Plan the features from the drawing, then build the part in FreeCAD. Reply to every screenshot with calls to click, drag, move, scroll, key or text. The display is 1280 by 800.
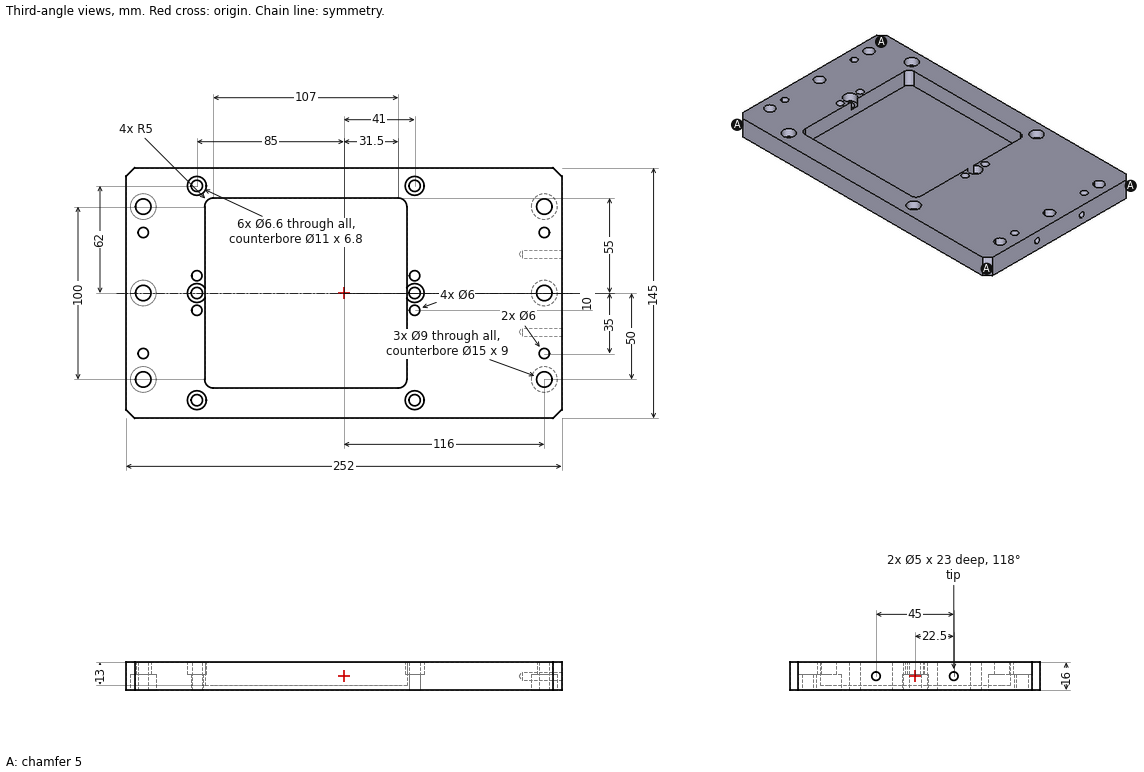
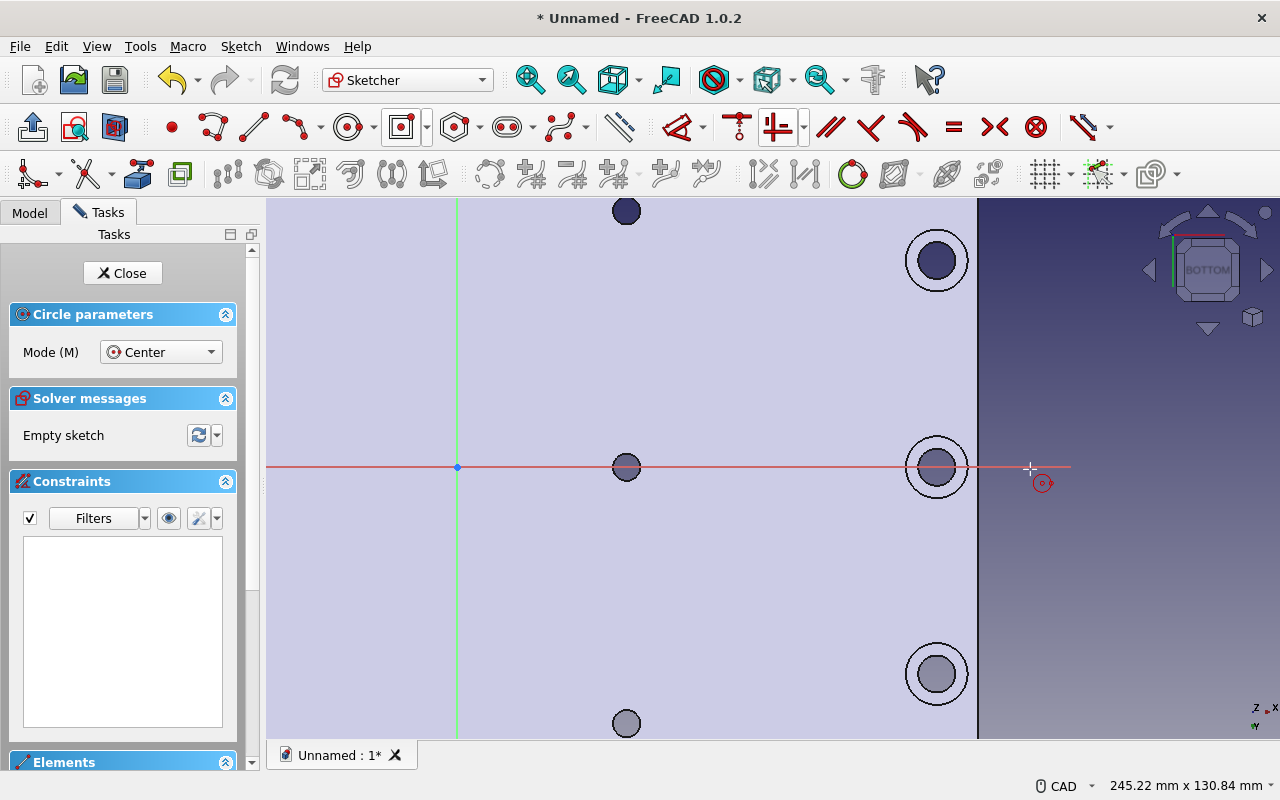
scroll(937, 323, up, 4)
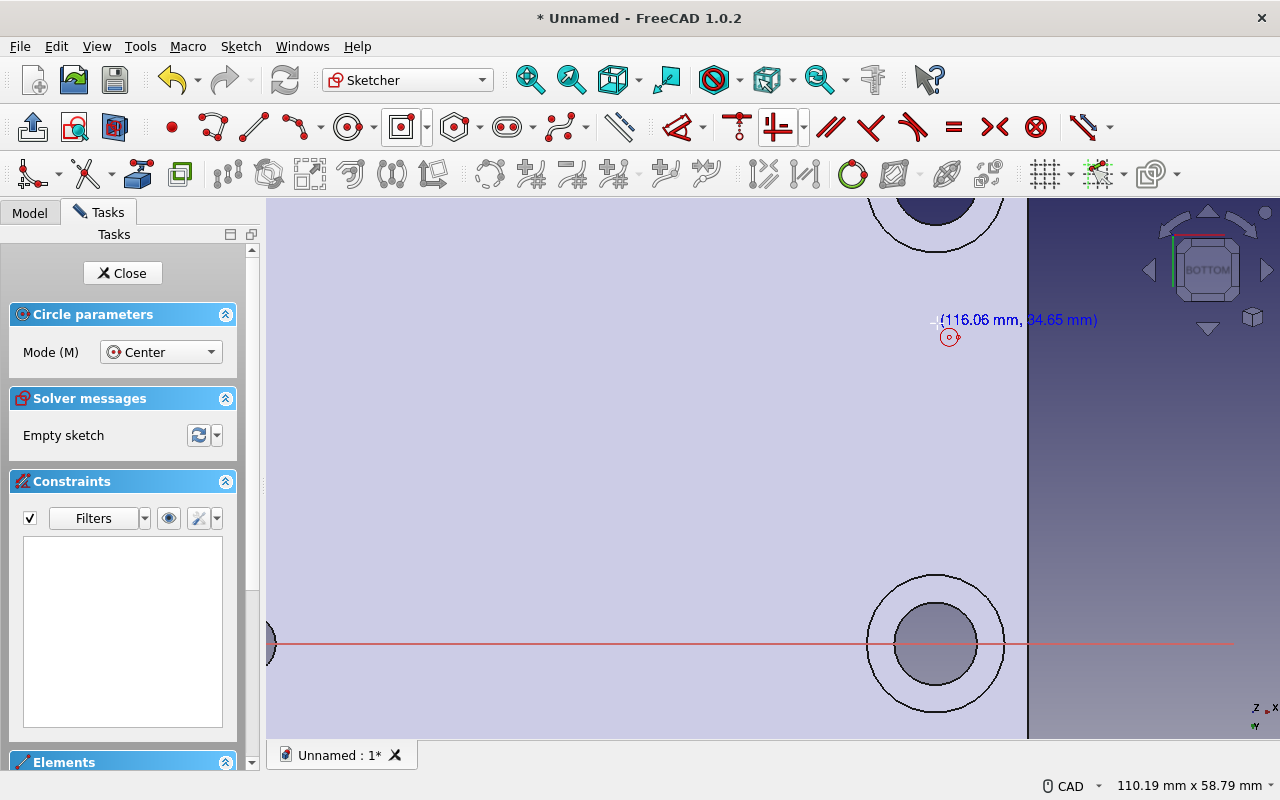
click(936, 322)
move(955, 302)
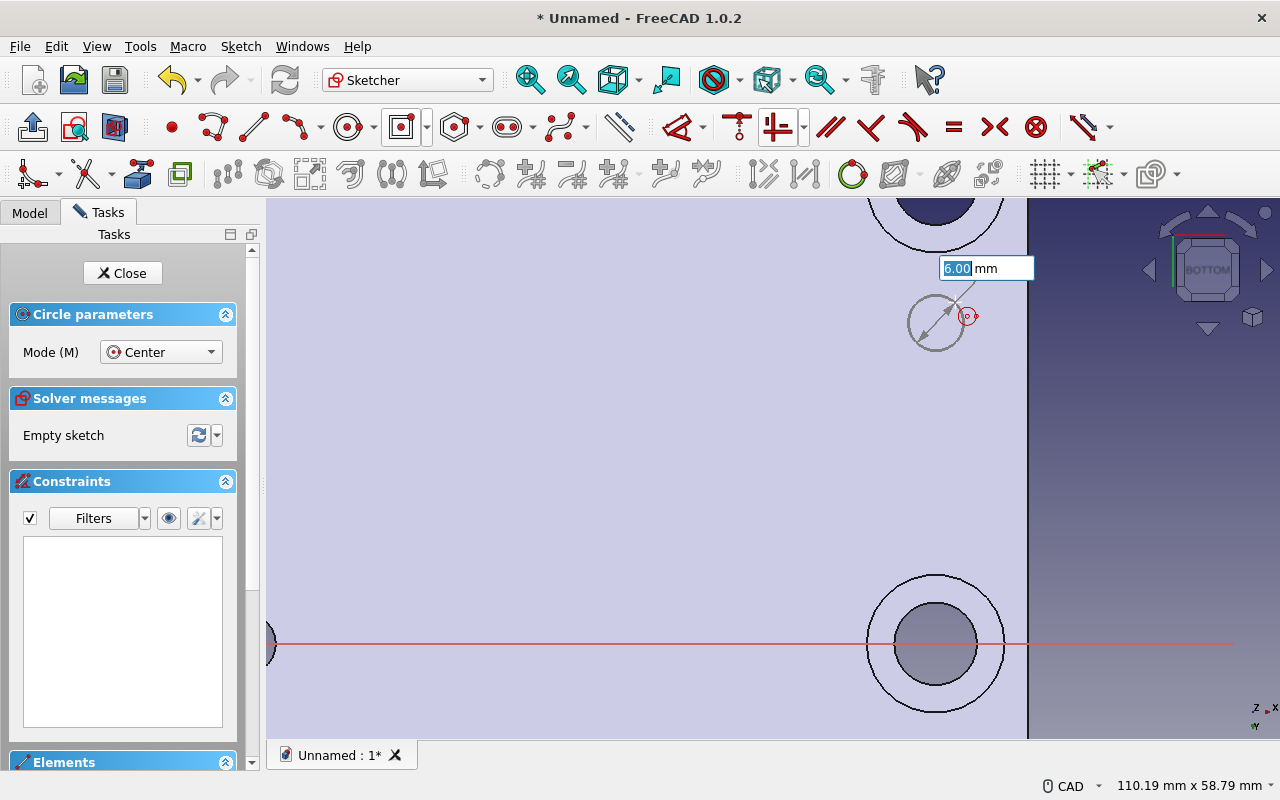
text(6)
key(Return)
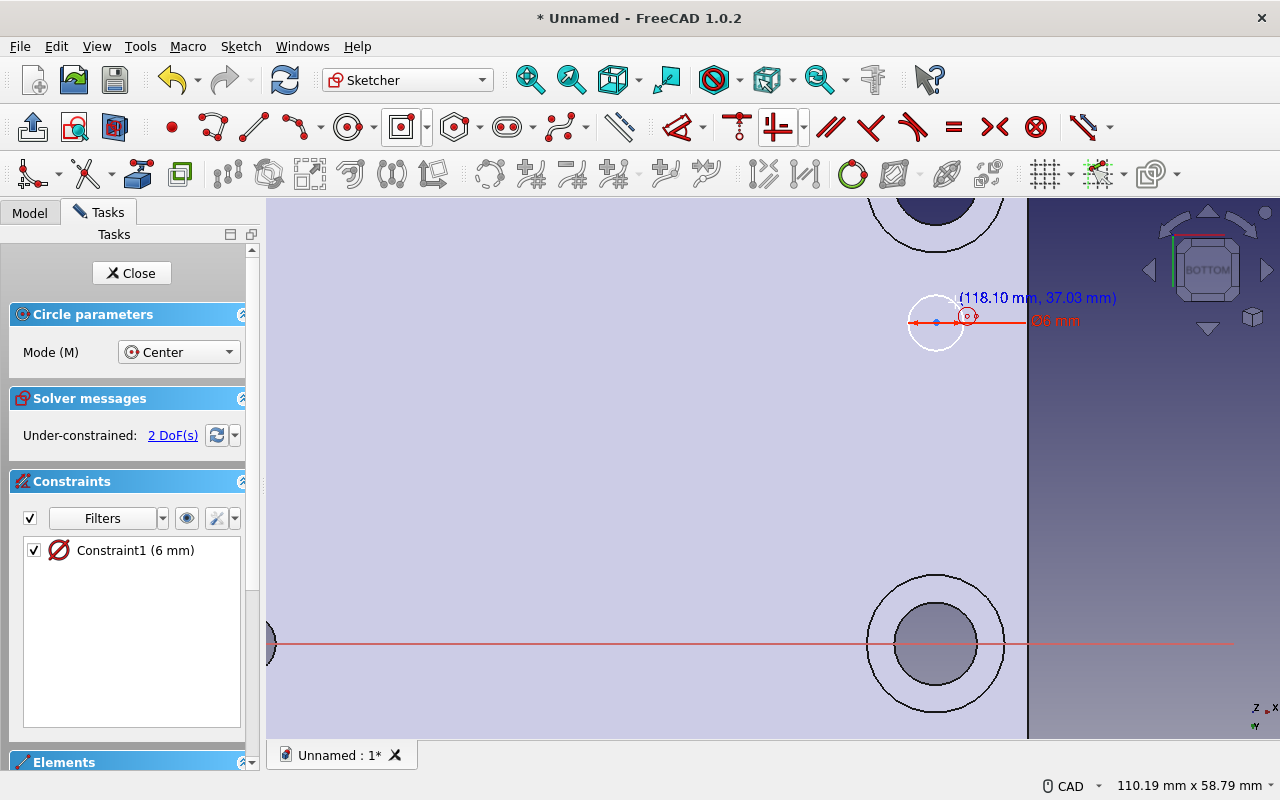
scroll(940, 325, down, 4)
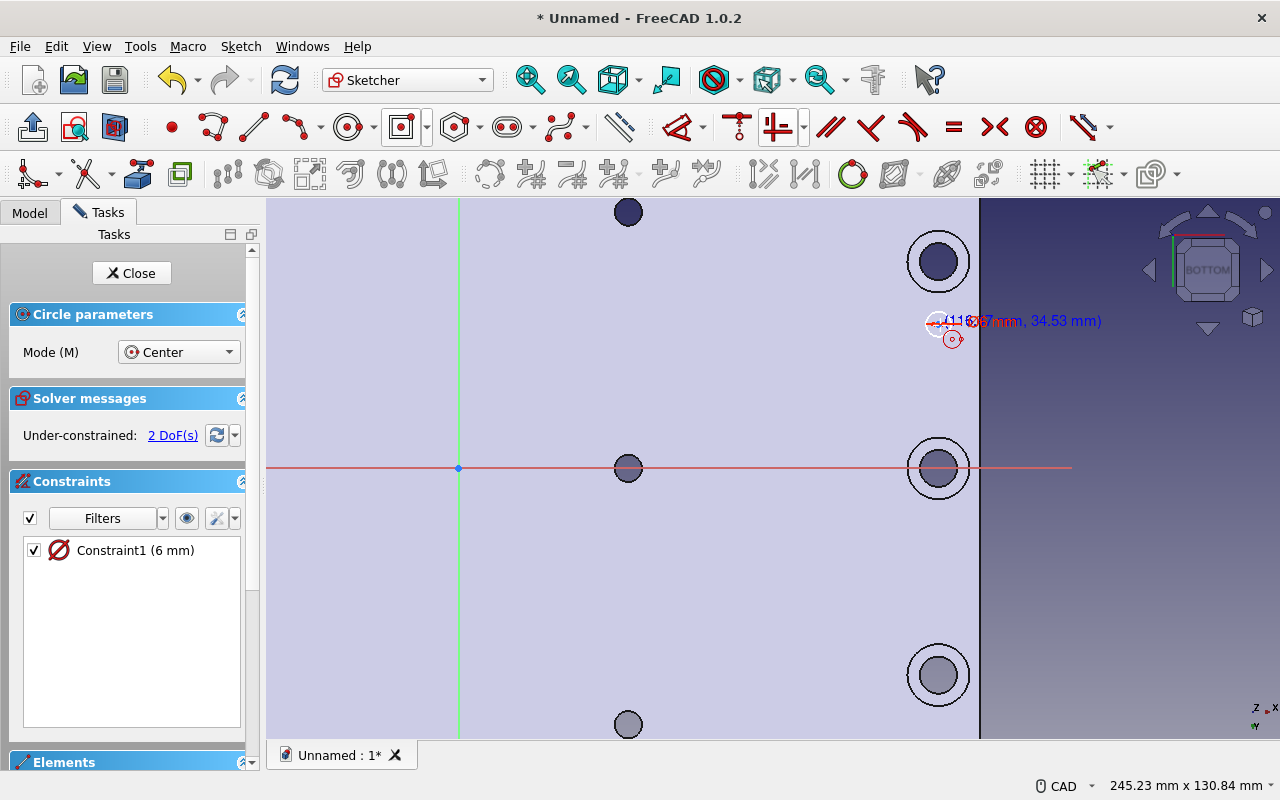
scroll(938, 613, up, 4)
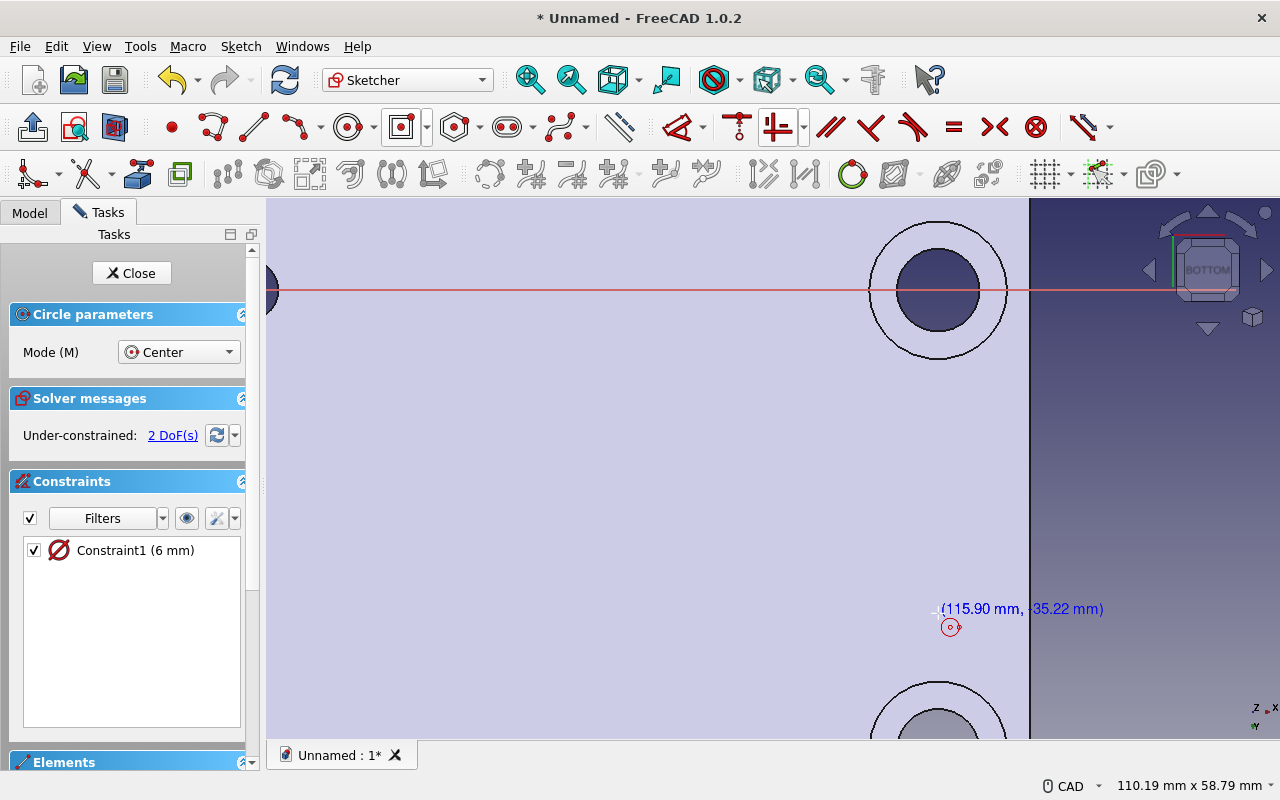
click(938, 612)
move(958, 593)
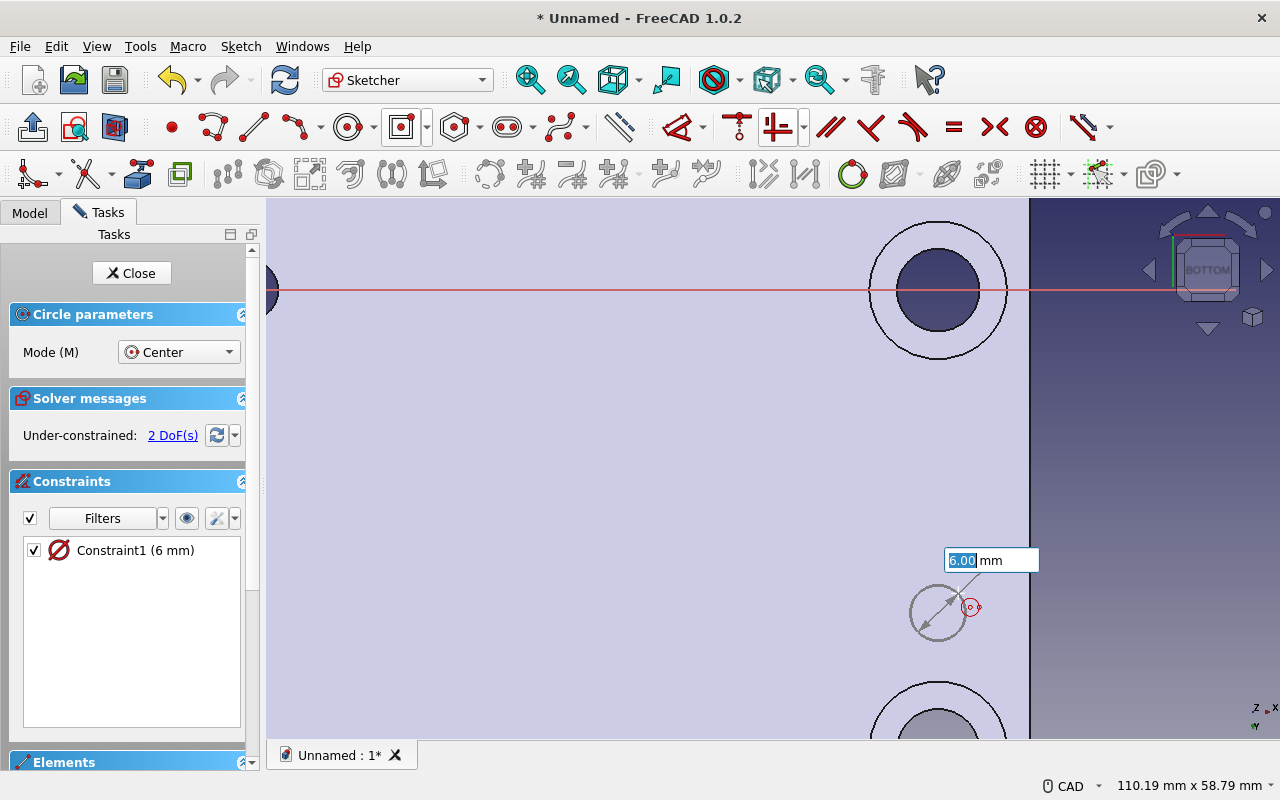
text(6)
key(Return)
key(Escape)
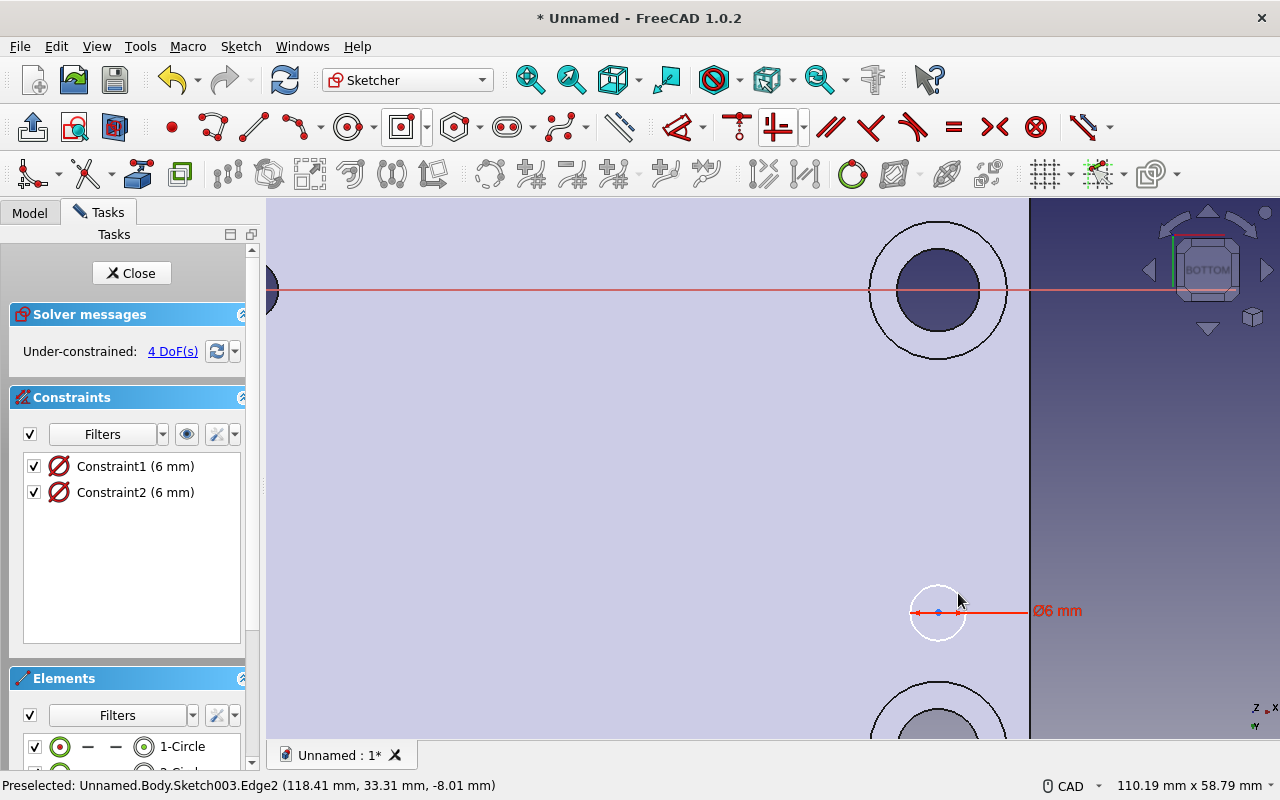
scroll(938, 614, down, 4)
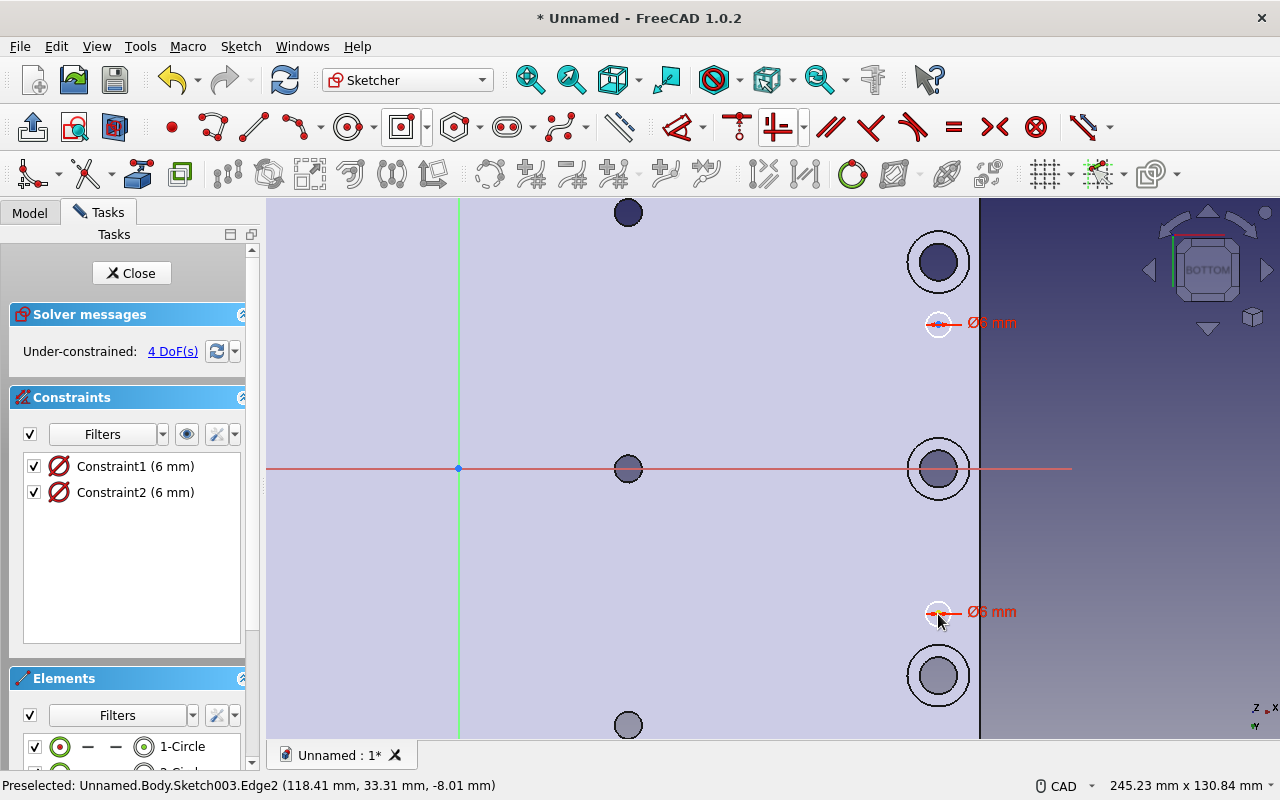
click(939, 325)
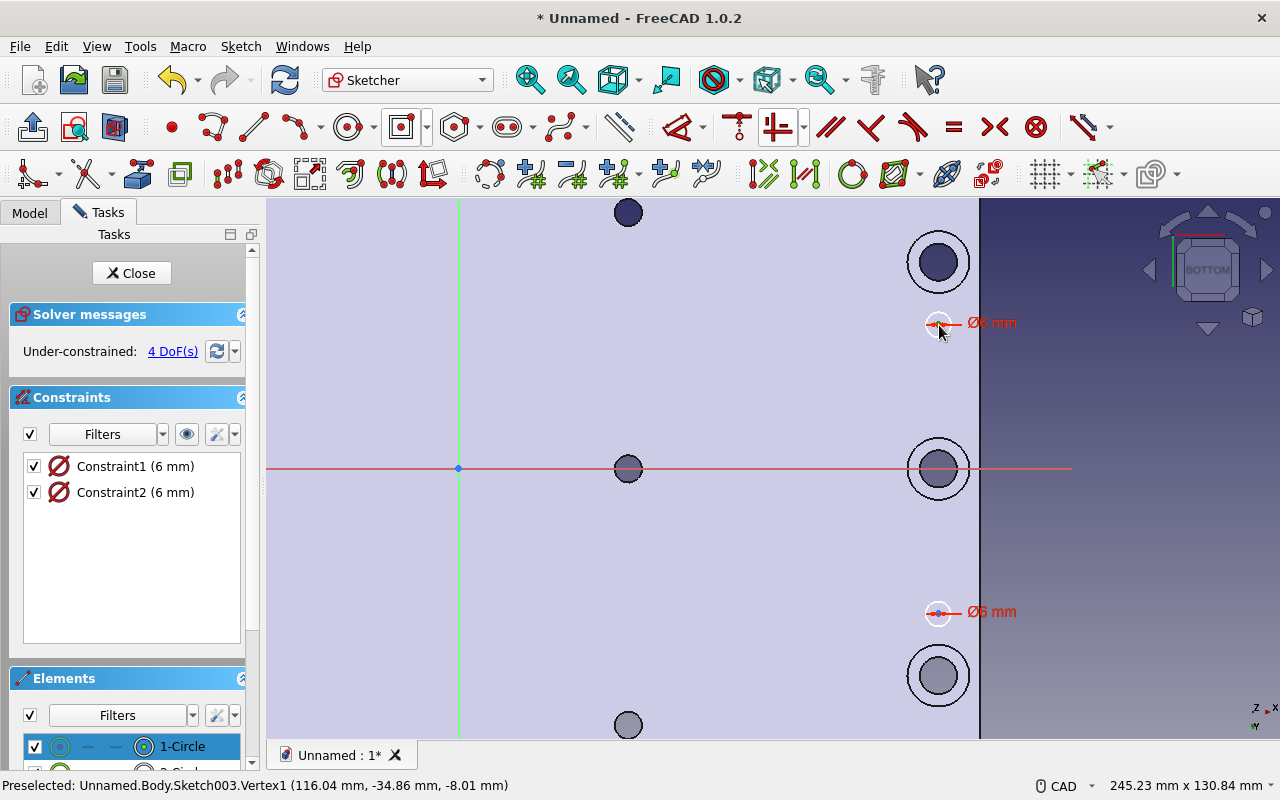
click(938, 614)